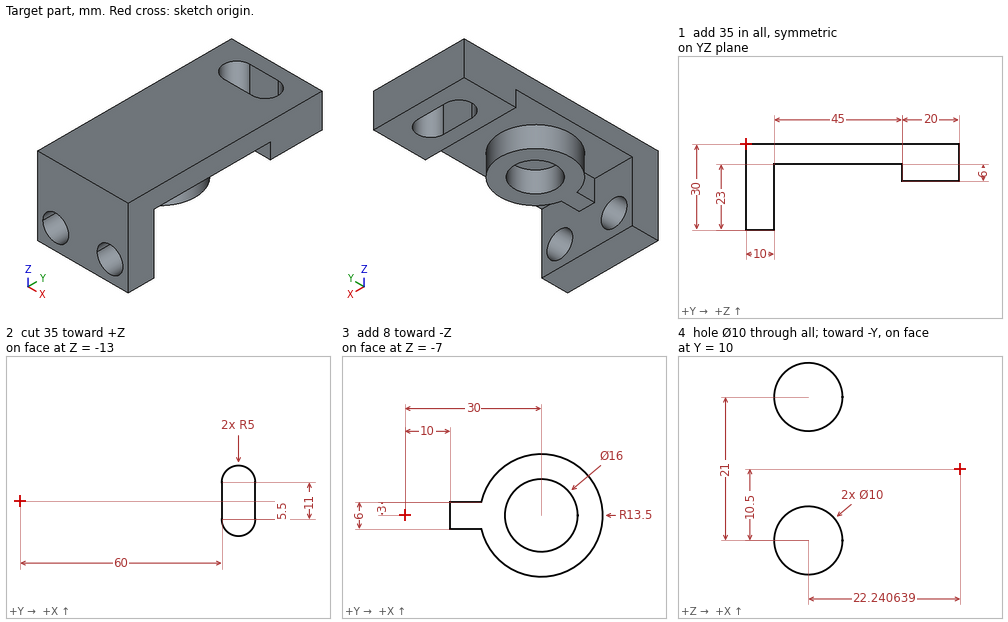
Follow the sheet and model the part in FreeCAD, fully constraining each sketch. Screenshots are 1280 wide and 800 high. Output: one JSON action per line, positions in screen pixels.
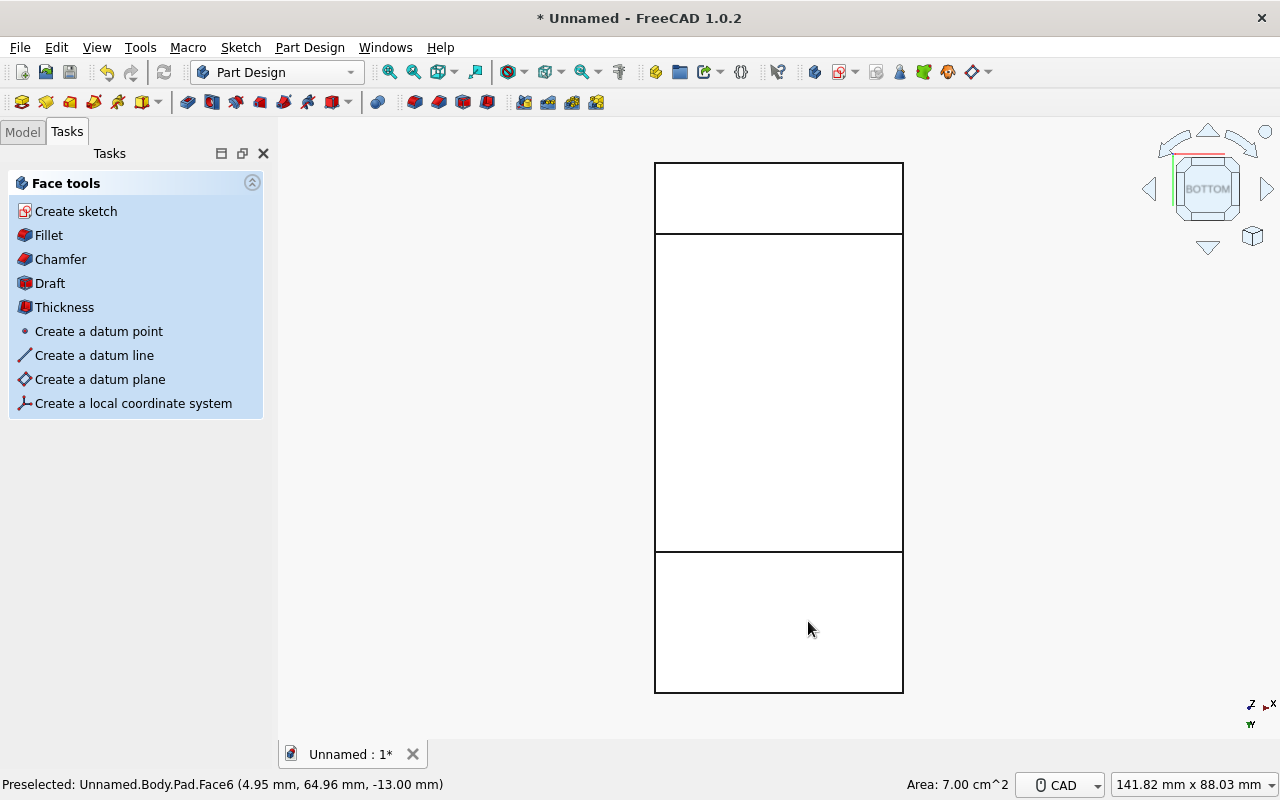
{"action": "left_click", "coordinate": [840, 72]}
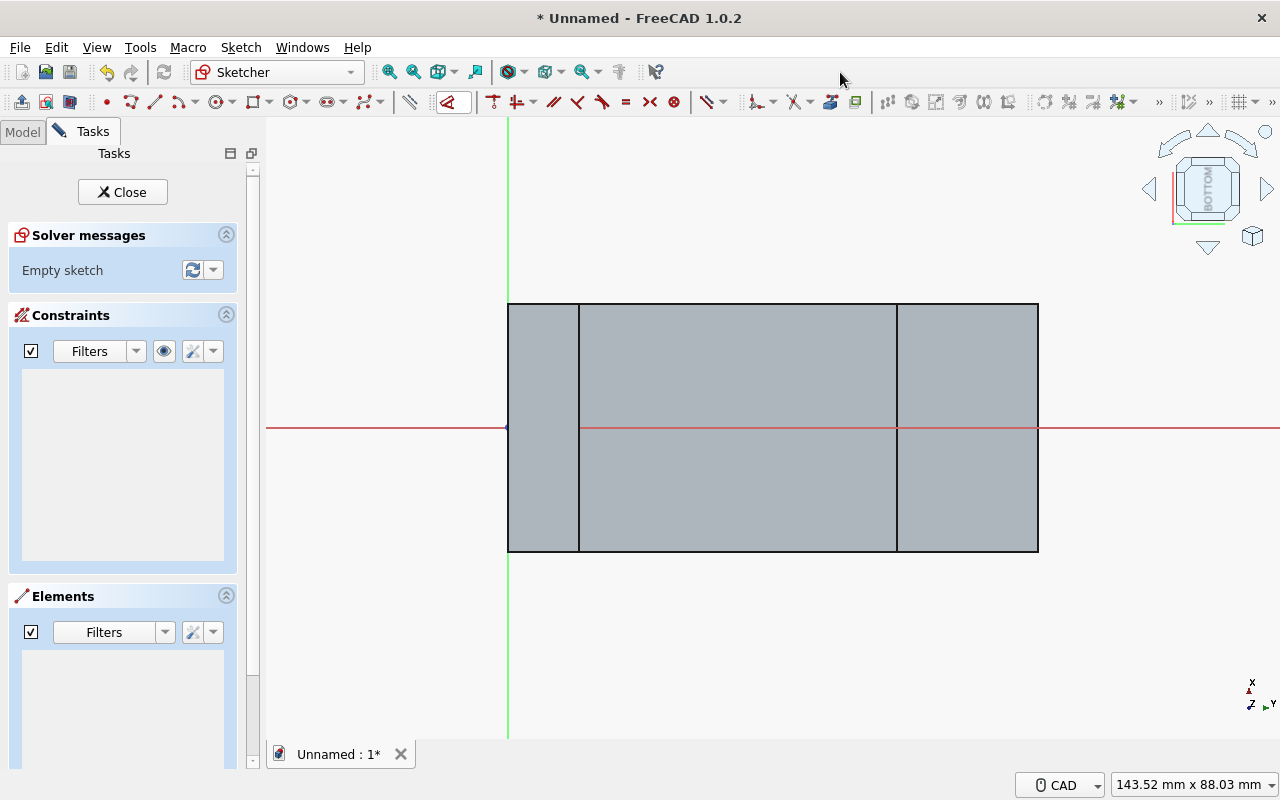
{"action": "scroll", "coordinate": [1115, 428], "scroll_direction": "up", "scroll_amount": 5}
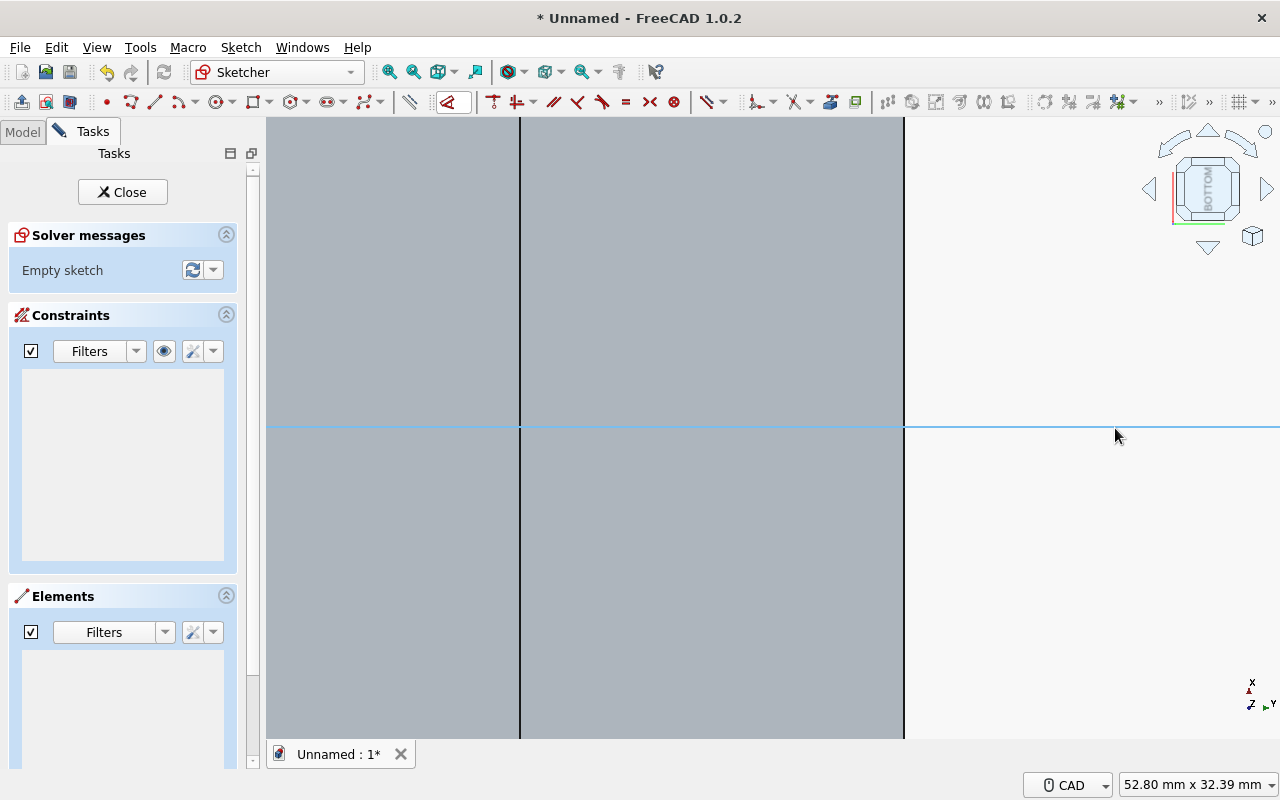
{"action": "left_click", "coordinate": [328, 102]}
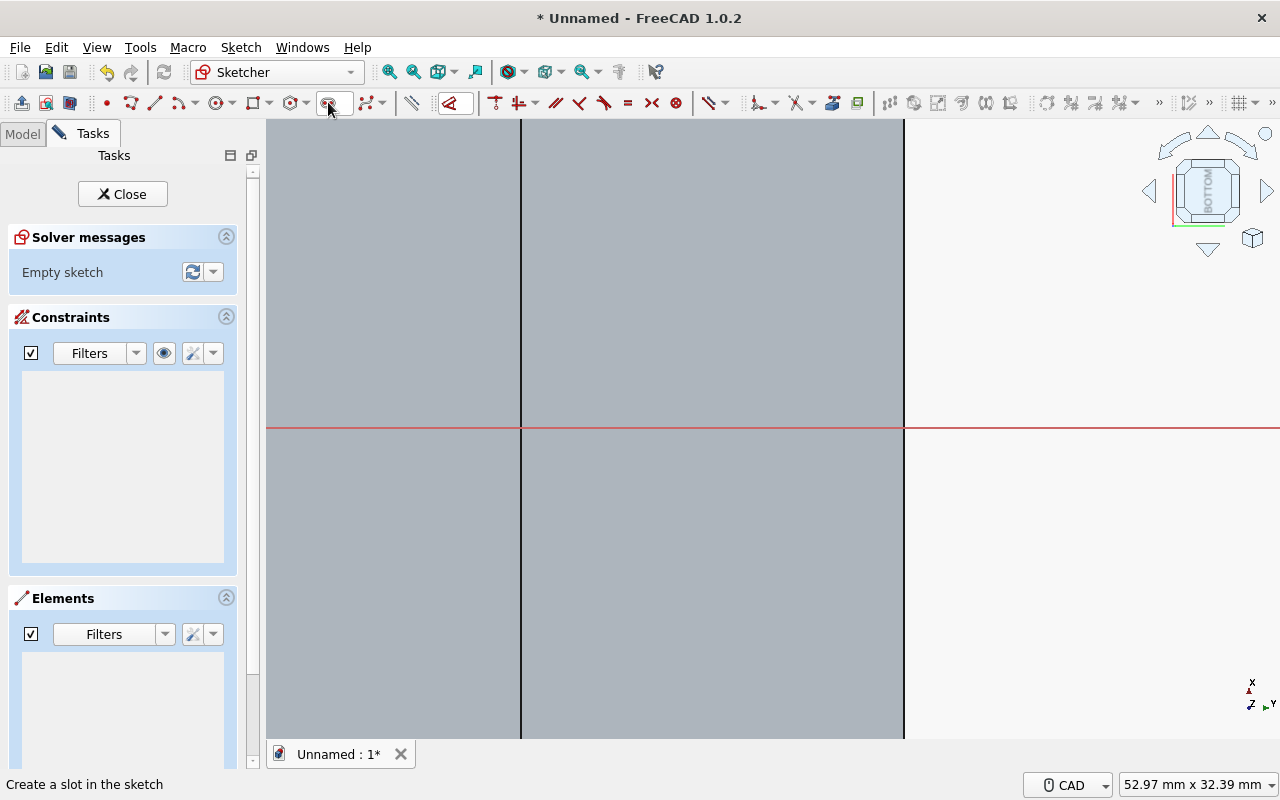
{"action": "left_click", "coordinate": [712, 533]}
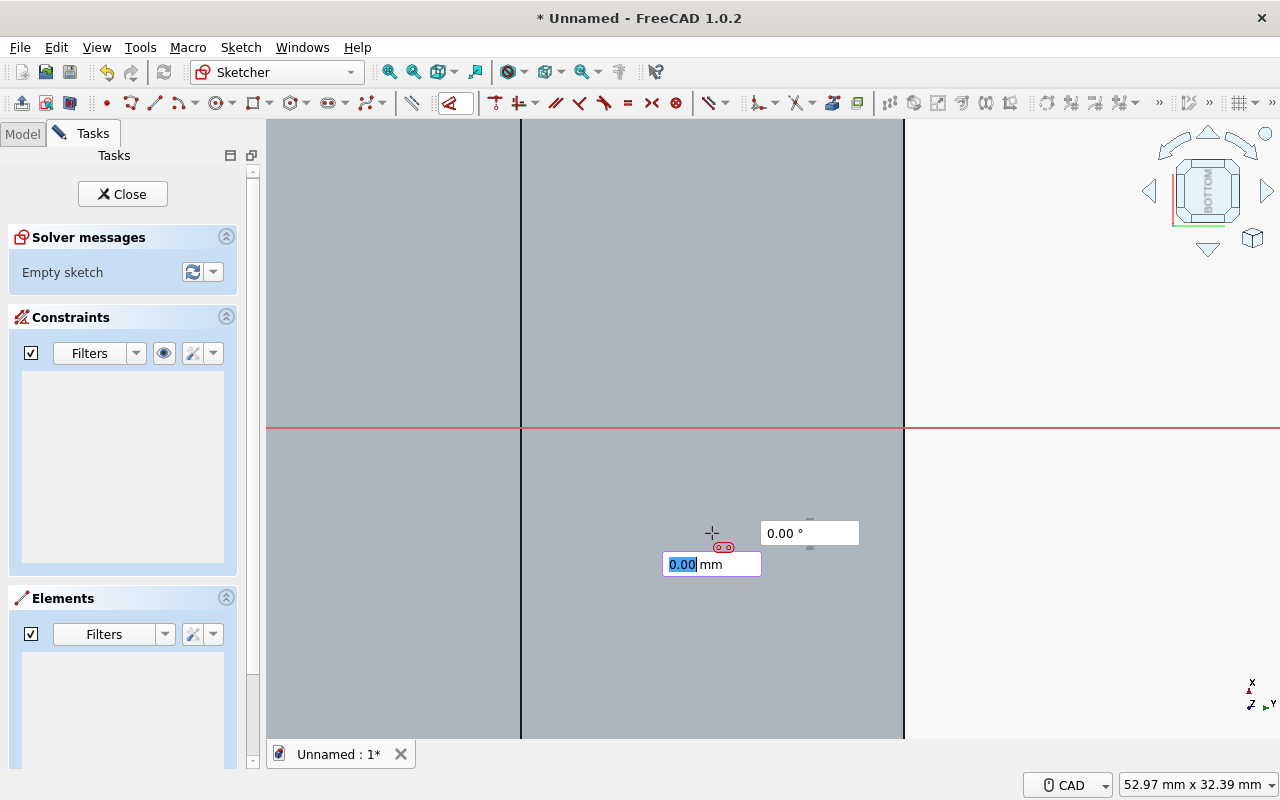
{"action": "left_click", "coordinate": [712, 323]}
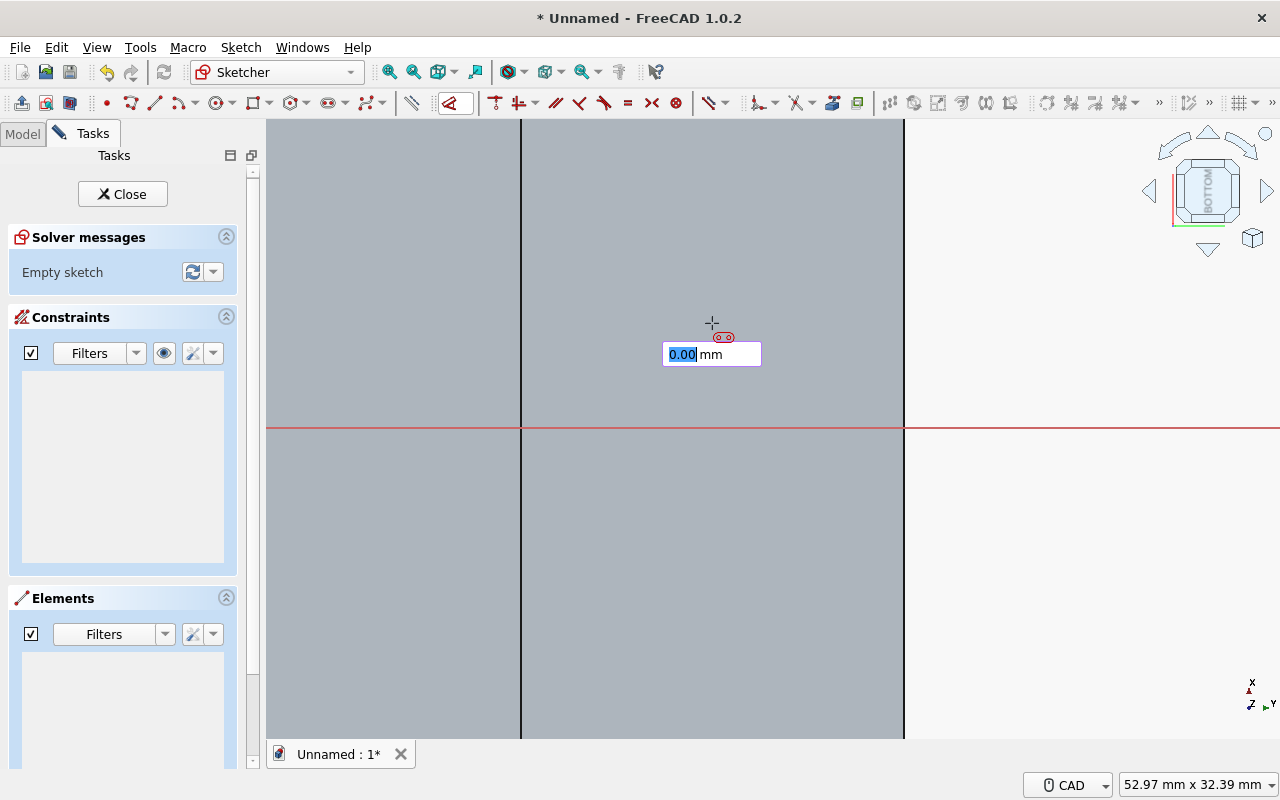
{"action": "left_click", "coordinate": [808, 460]}
{"action": "key", "text": "Escape"}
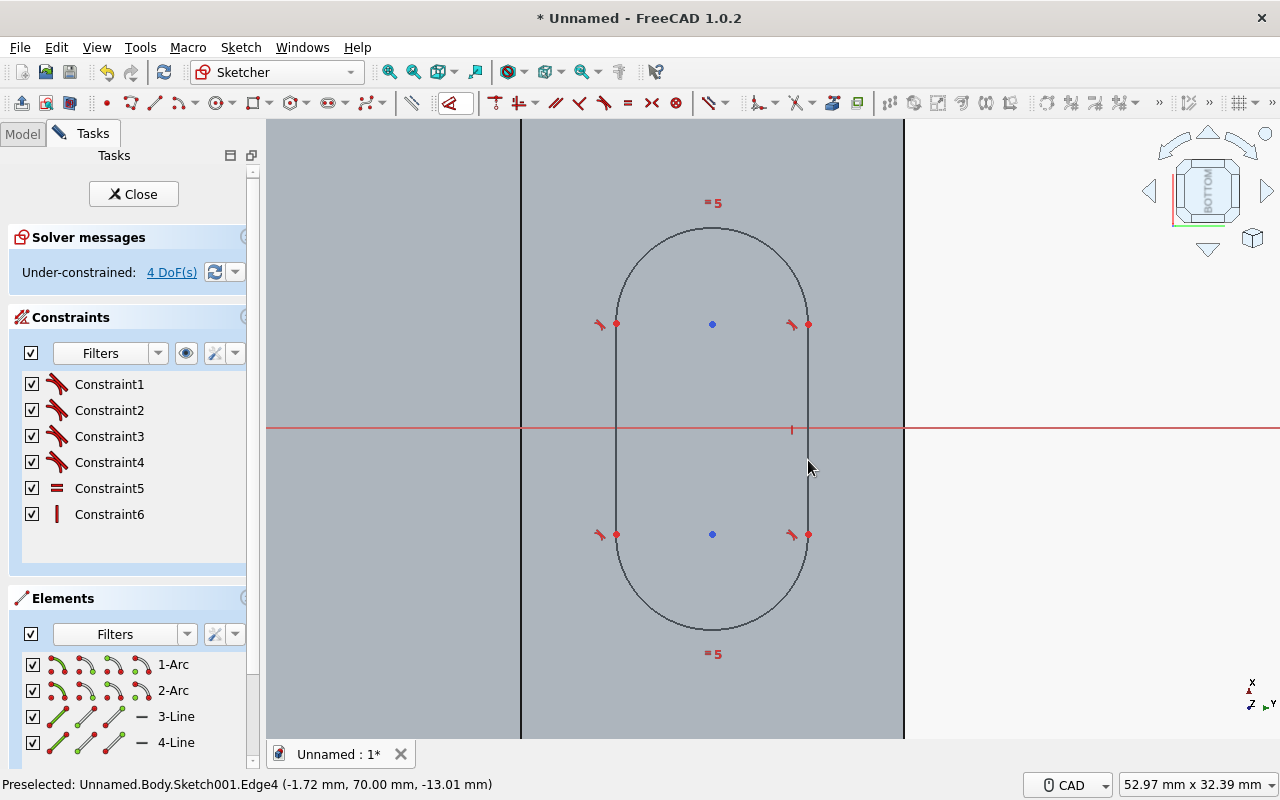
{"action": "left_click", "coordinate": [656, 612]}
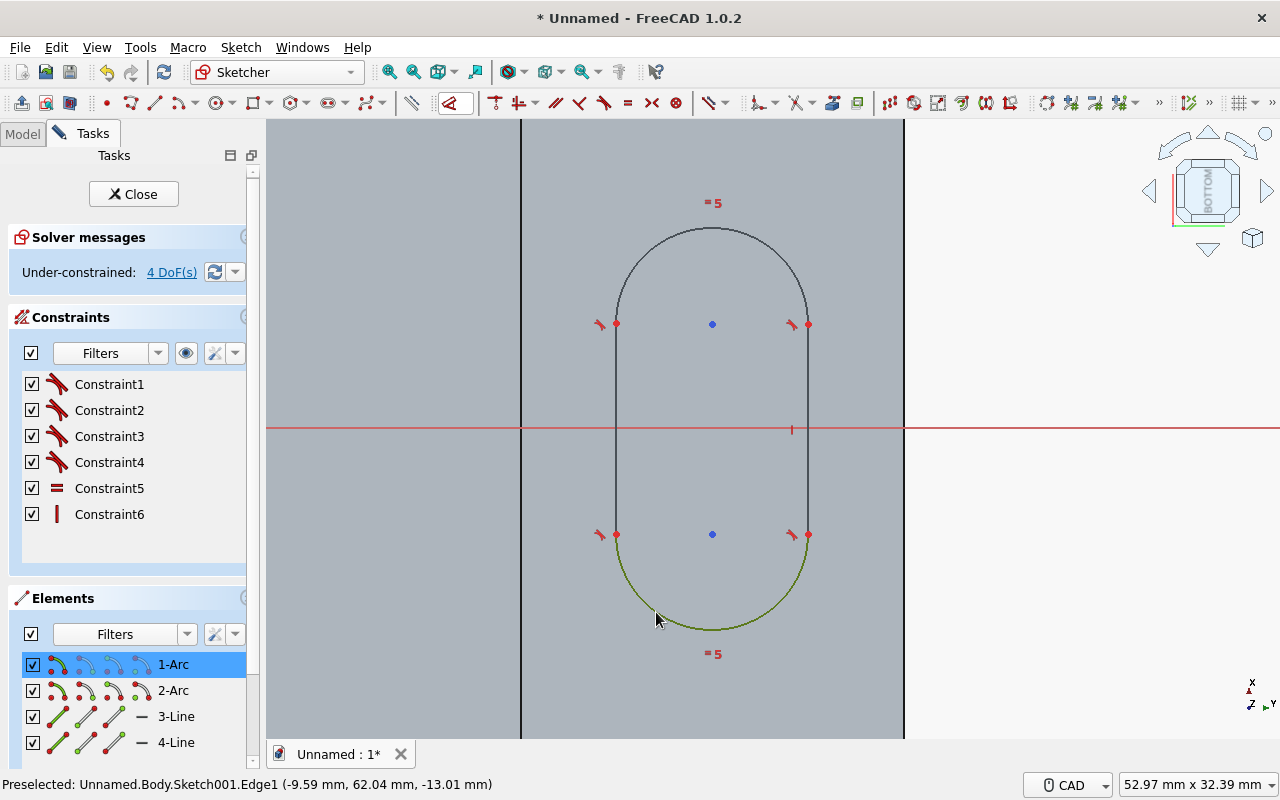
{"action": "key", "text": "k r"}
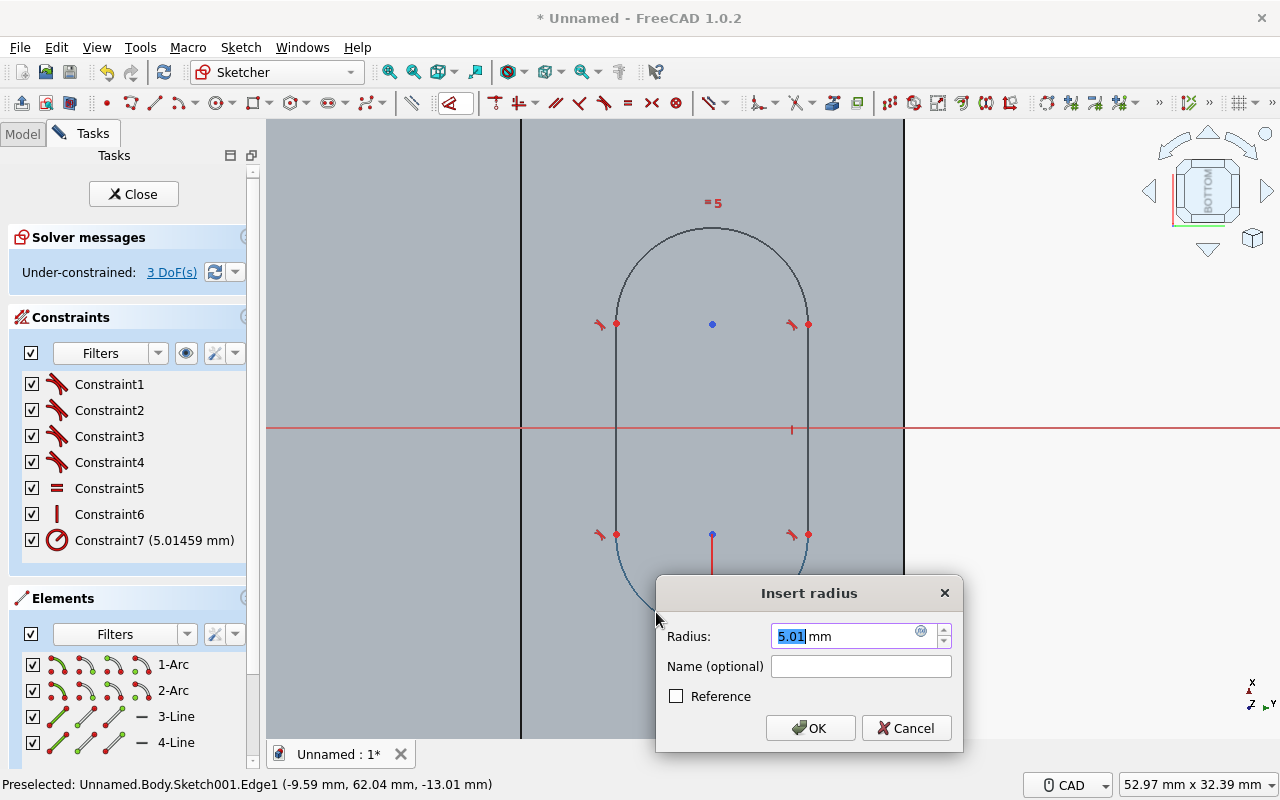
{"action": "type", "text": "5"}
{"action": "key", "text": "Return"}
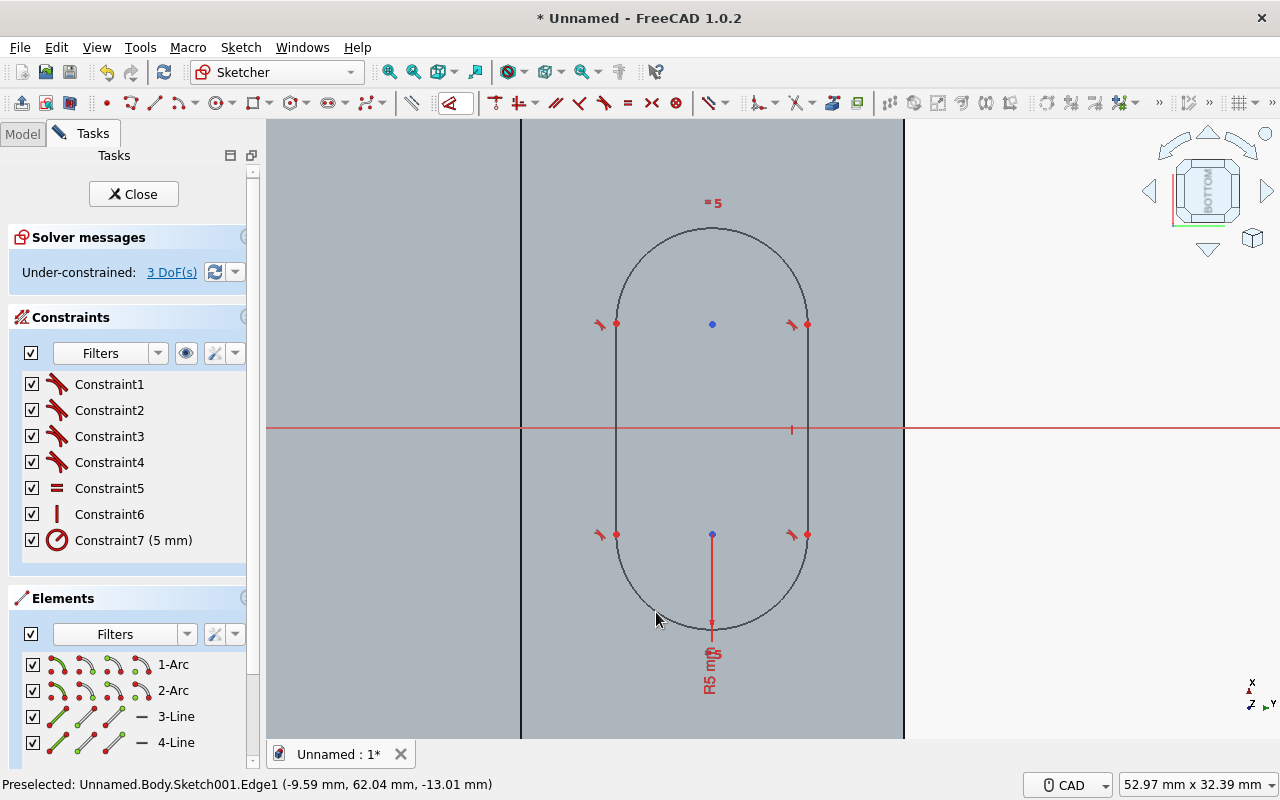
{"action": "left_click", "coordinate": [616, 471]}